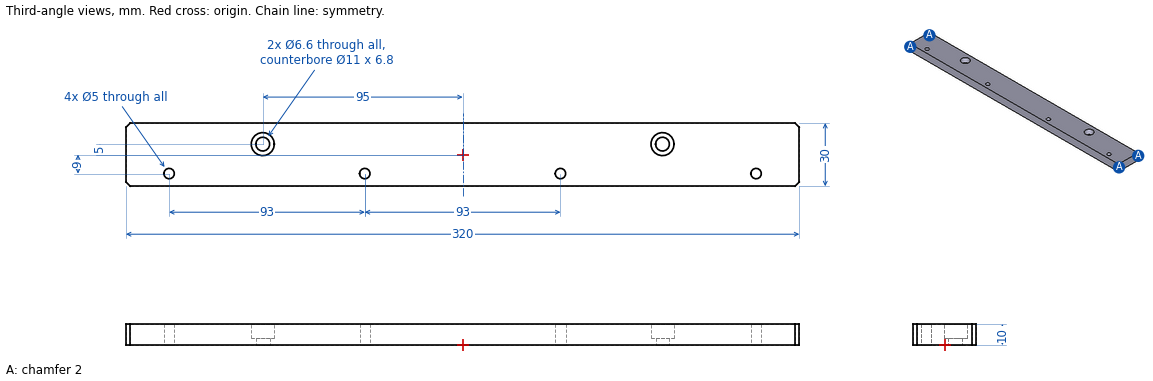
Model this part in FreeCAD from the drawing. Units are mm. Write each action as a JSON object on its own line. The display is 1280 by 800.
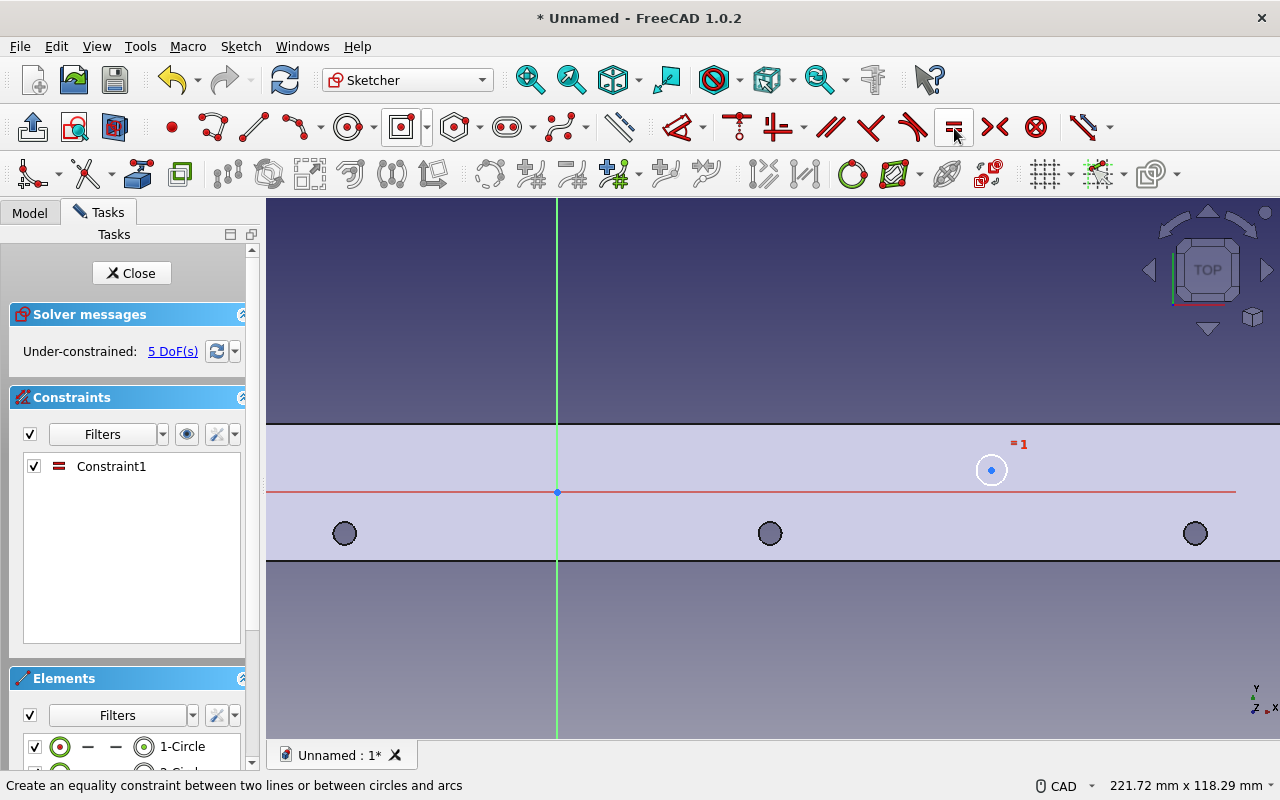
{"action": "scroll", "coordinate": [1003, 459], "scroll_direction": "down", "scroll_amount": 2}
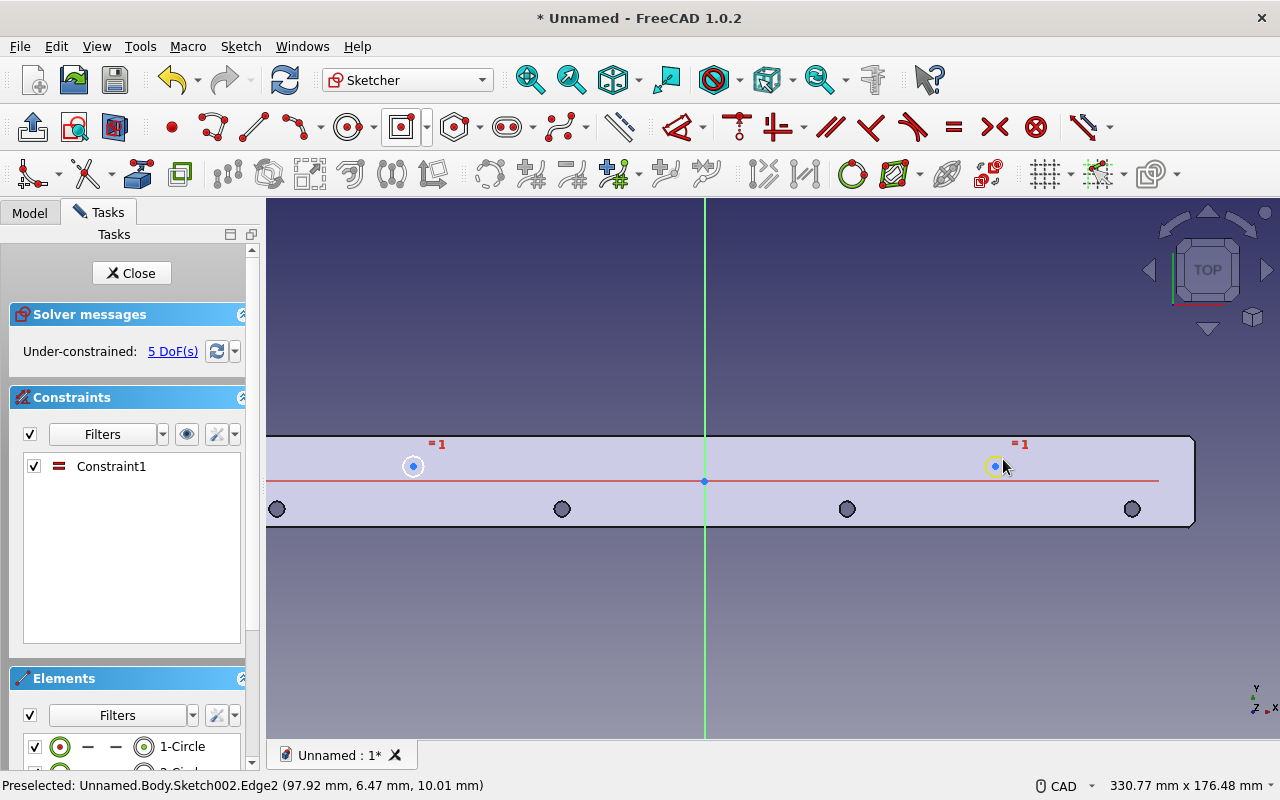
{"action": "left_click", "coordinate": [413, 467]}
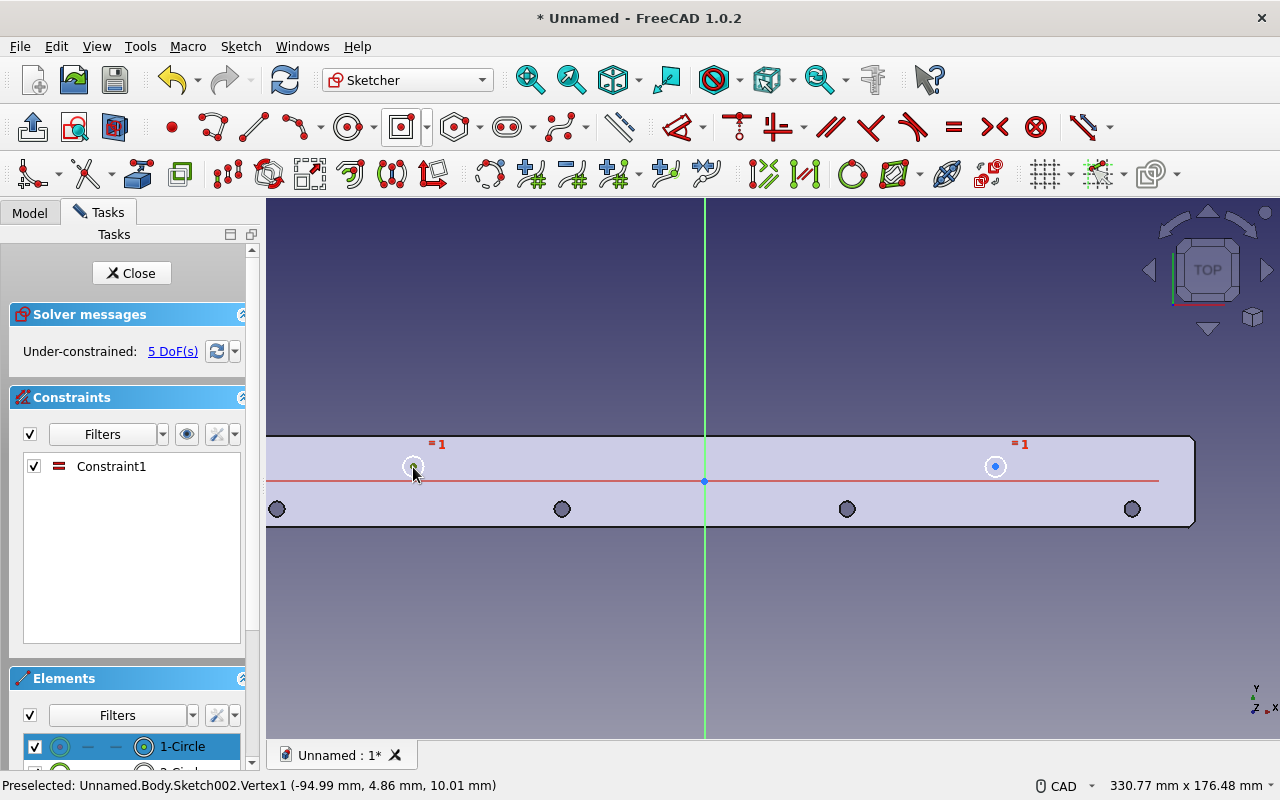
{"action": "left_click", "coordinate": [996, 467]}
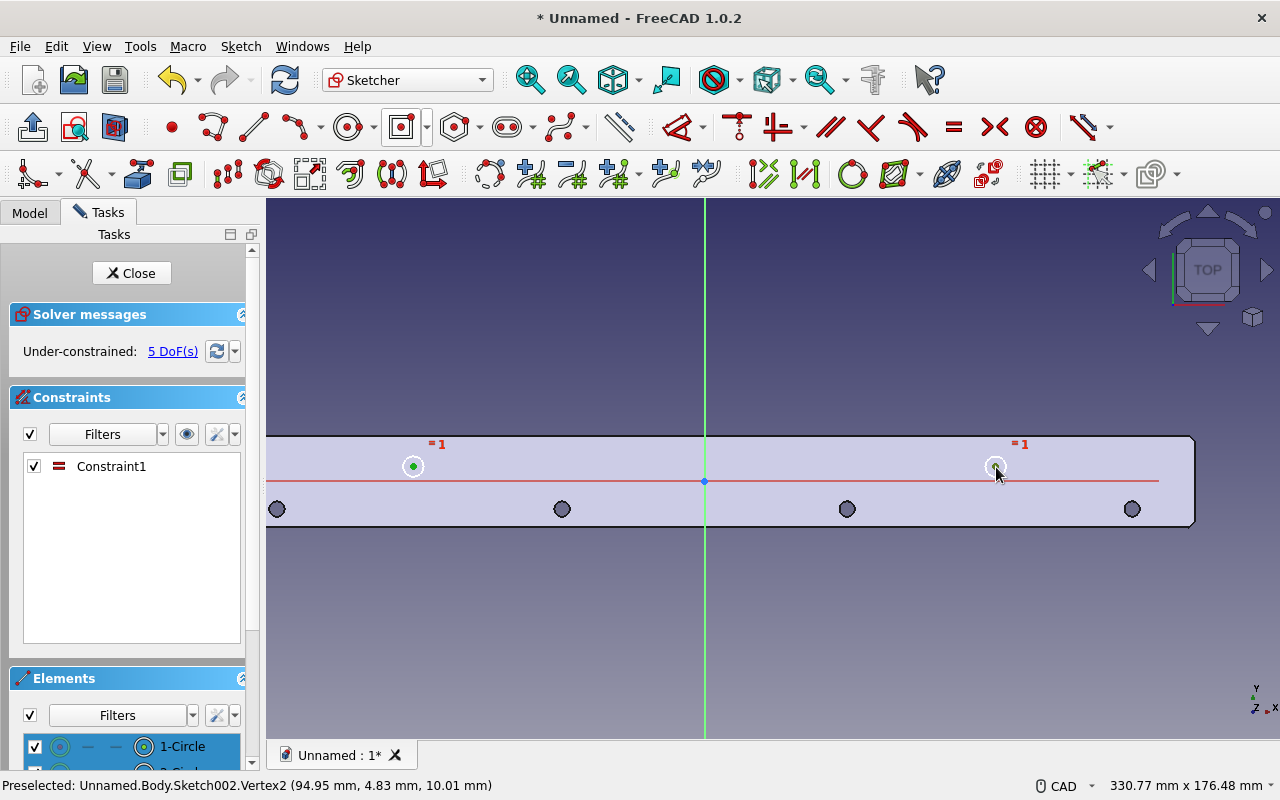
{"action": "left_click", "coordinate": [705, 676]}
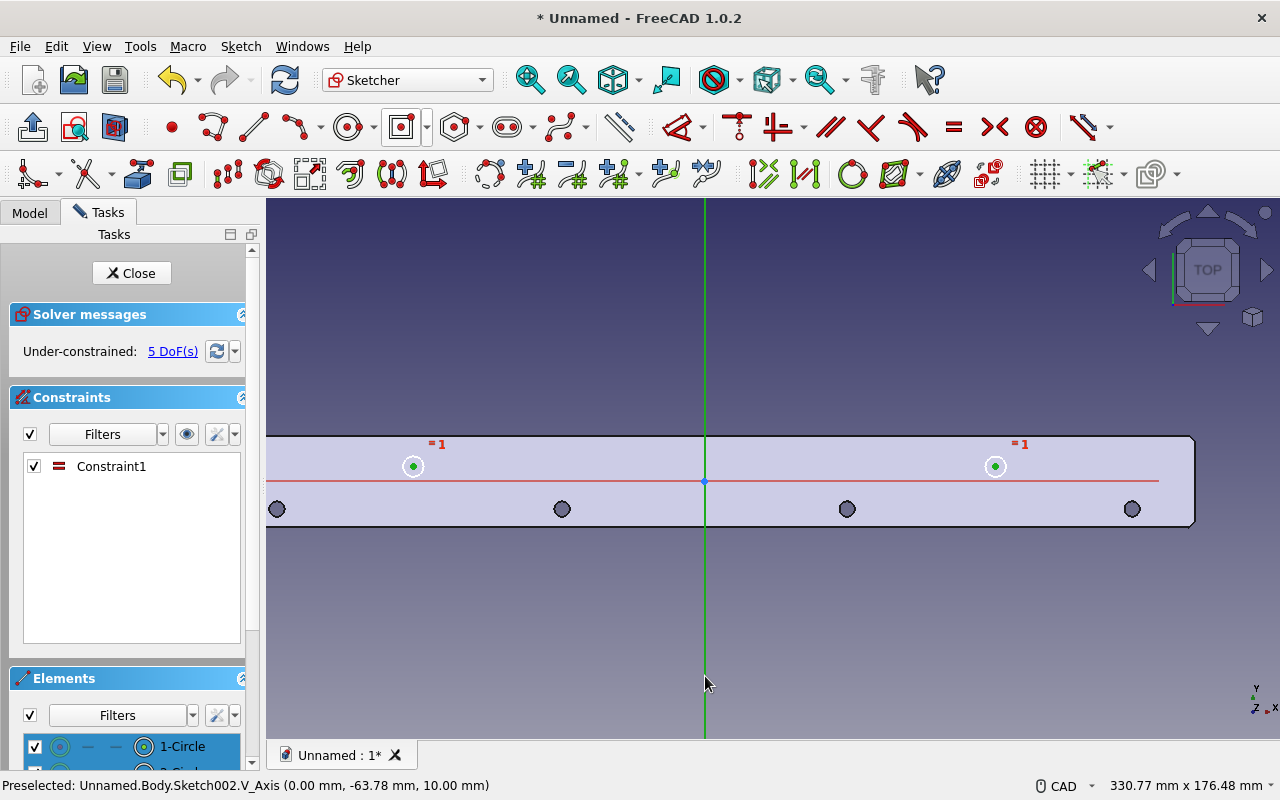
{"action": "left_click", "coordinate": [995, 128]}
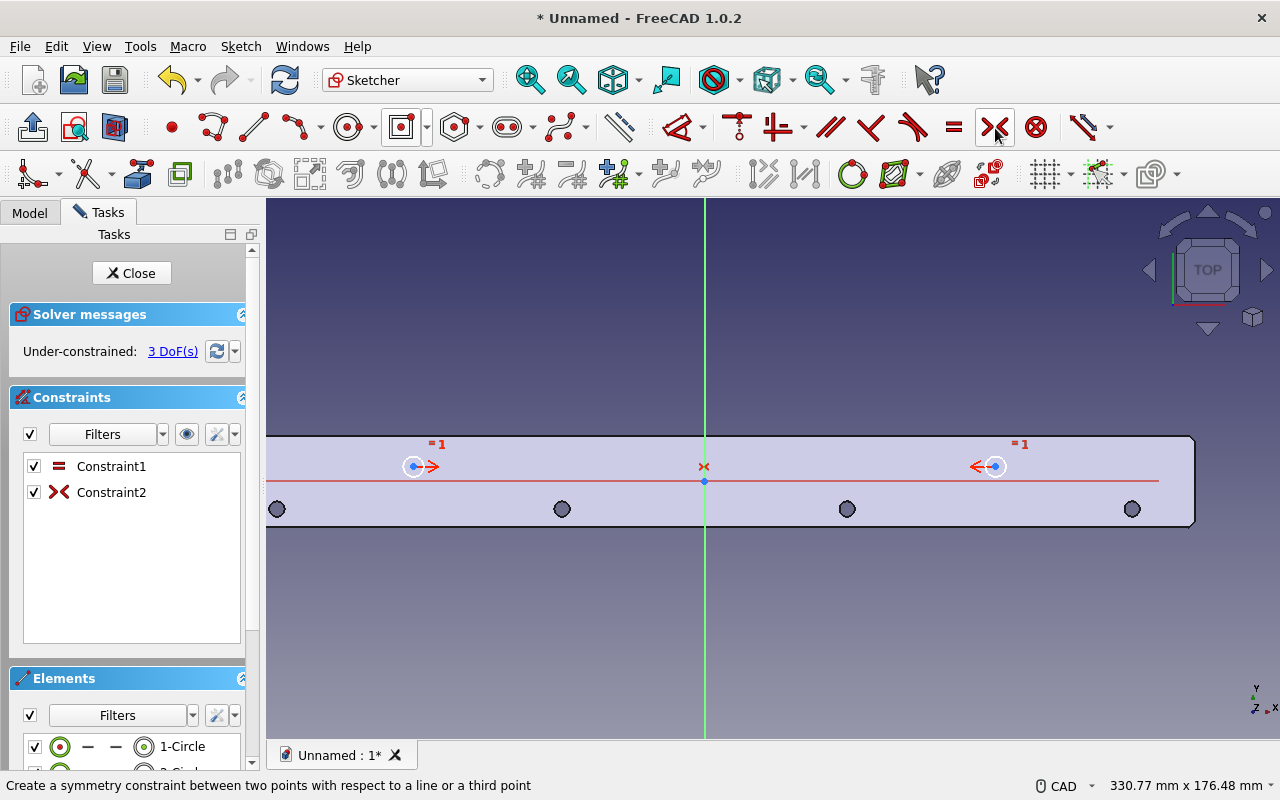
{"action": "left_click", "coordinate": [676, 128]}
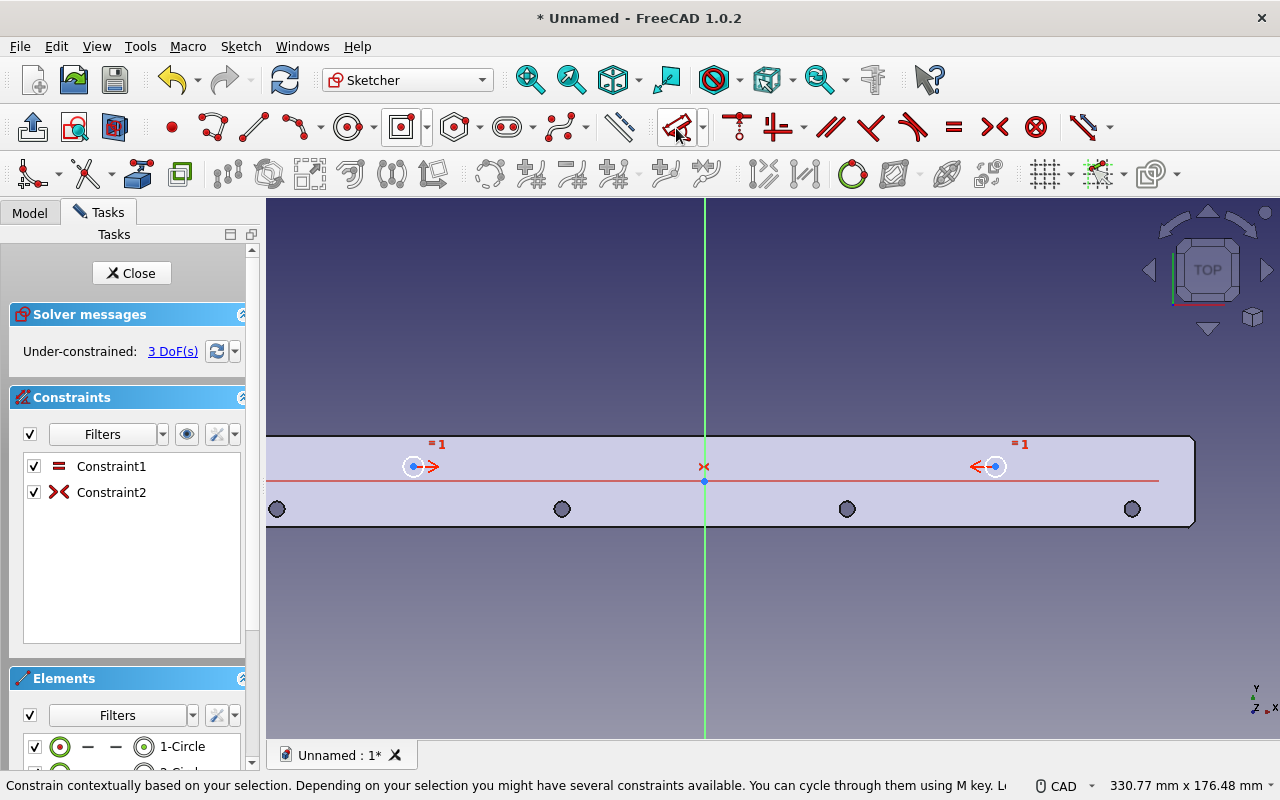
{"action": "scroll", "coordinate": [421, 459], "scroll_direction": "up", "scroll_amount": 4}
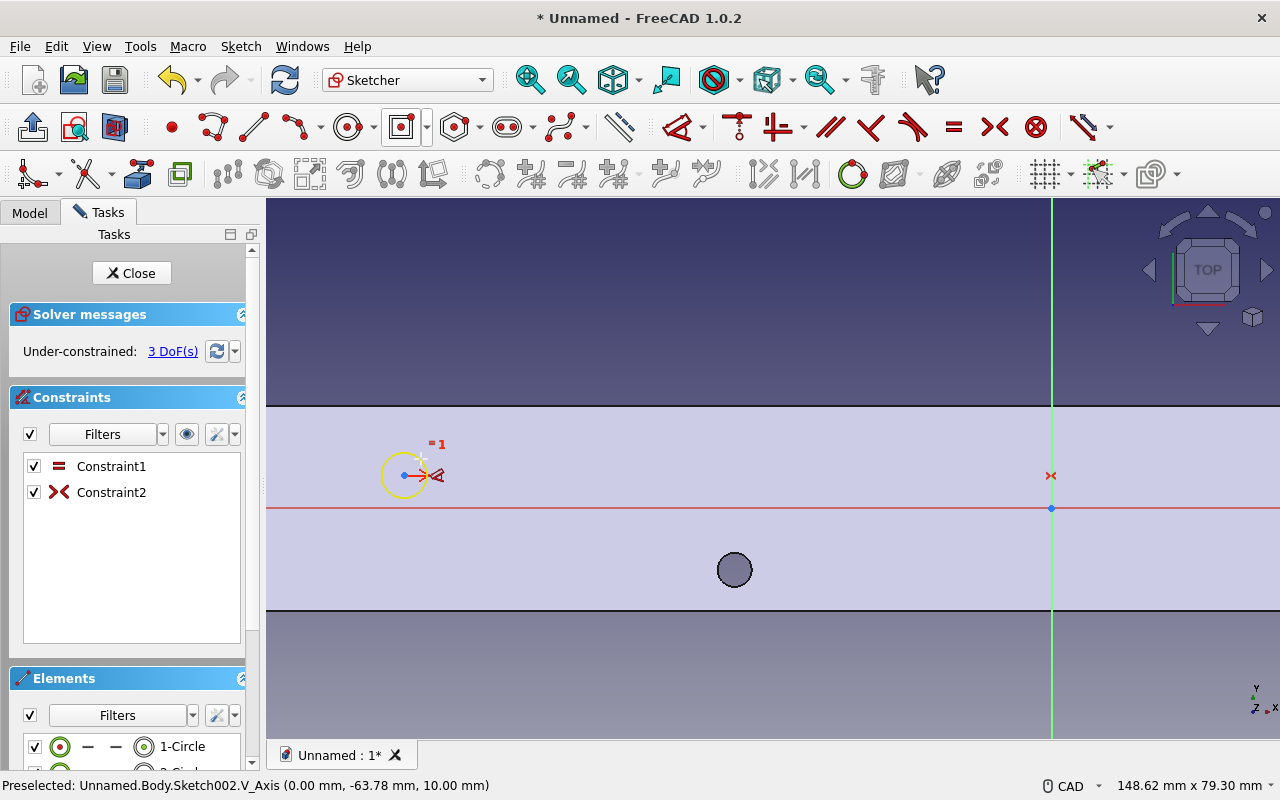
{"action": "left_click", "coordinate": [420, 459]}
{"action": "left_click", "coordinate": [442, 436]}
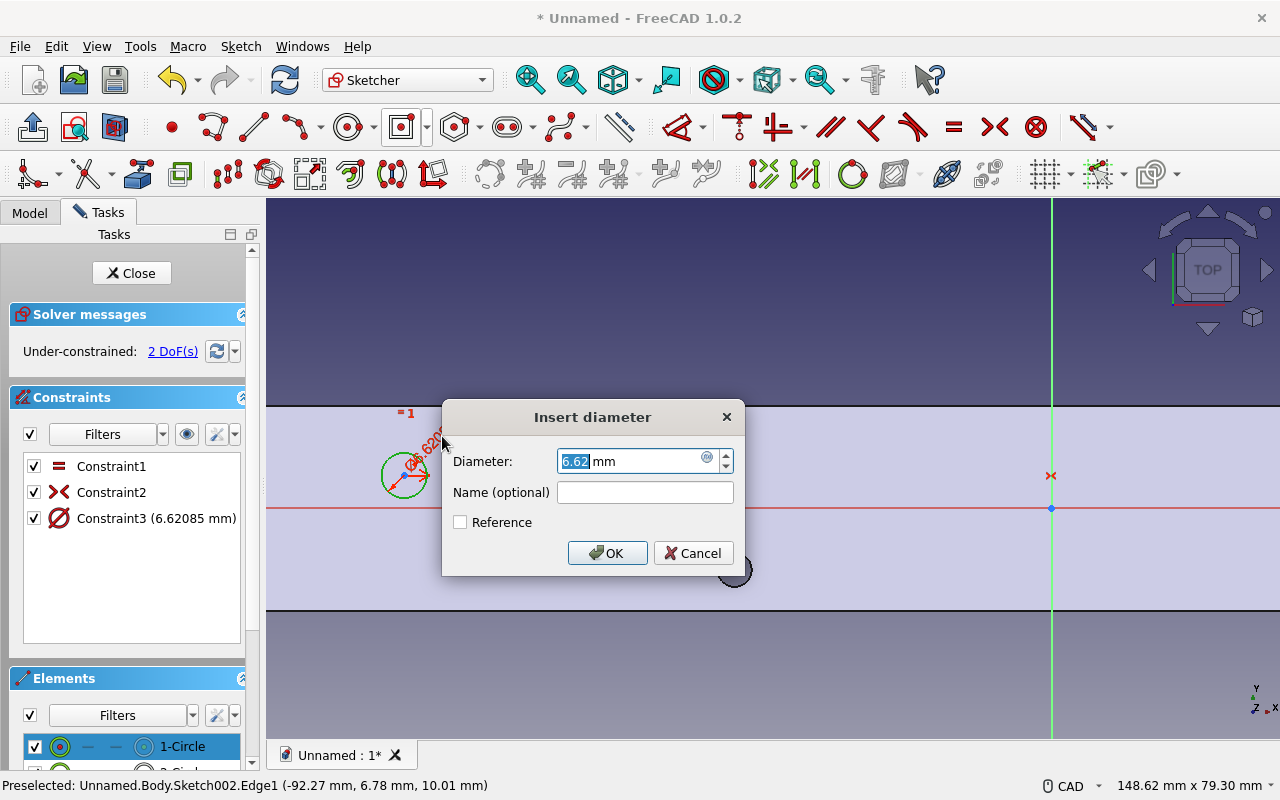
{"action": "type", "text": "6.6"}
{"action": "key", "text": "Return"}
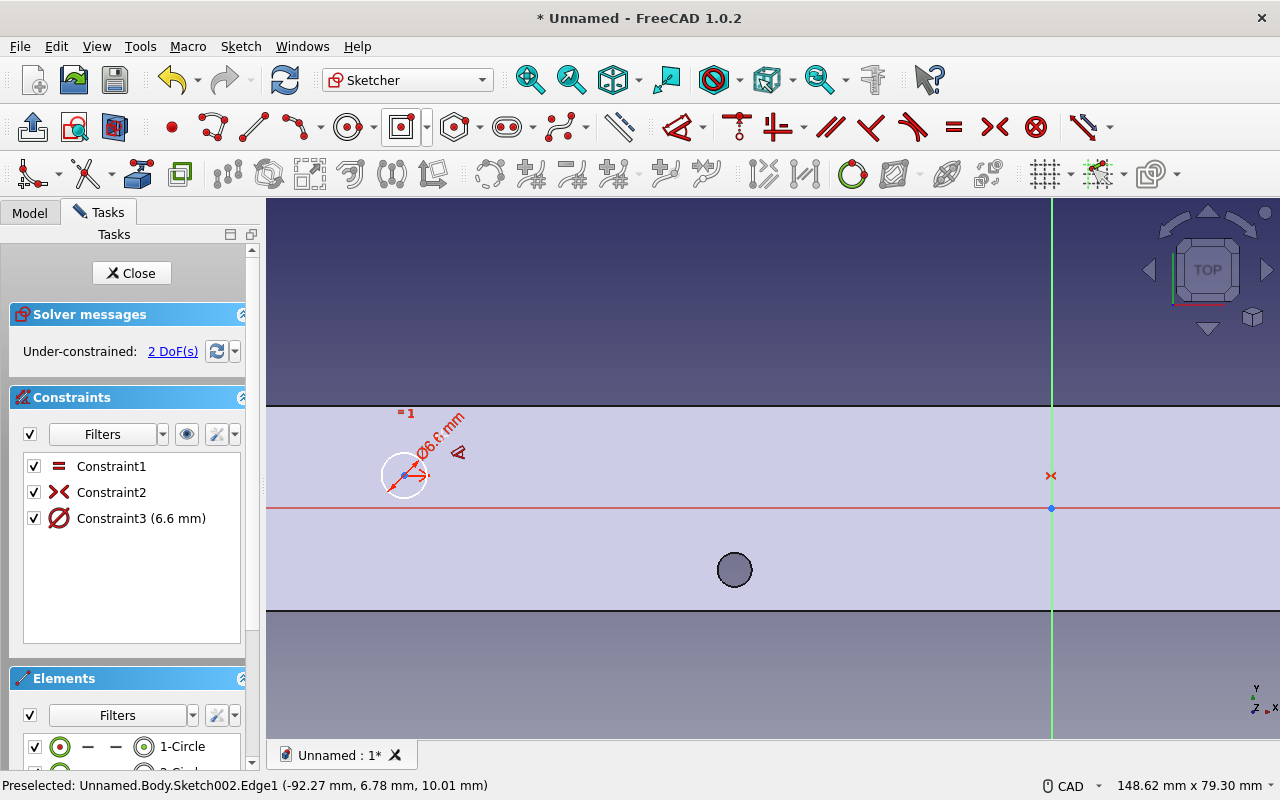
{"action": "left_click", "coordinate": [404, 476]}
{"action": "left_click", "coordinate": [370, 492]}